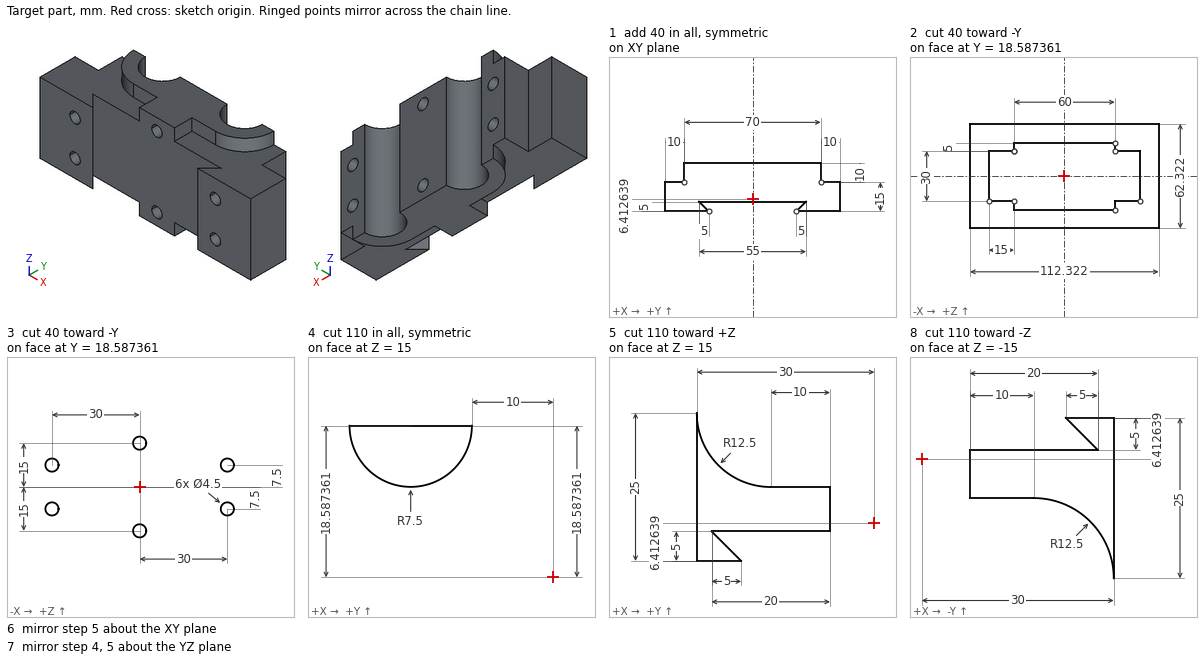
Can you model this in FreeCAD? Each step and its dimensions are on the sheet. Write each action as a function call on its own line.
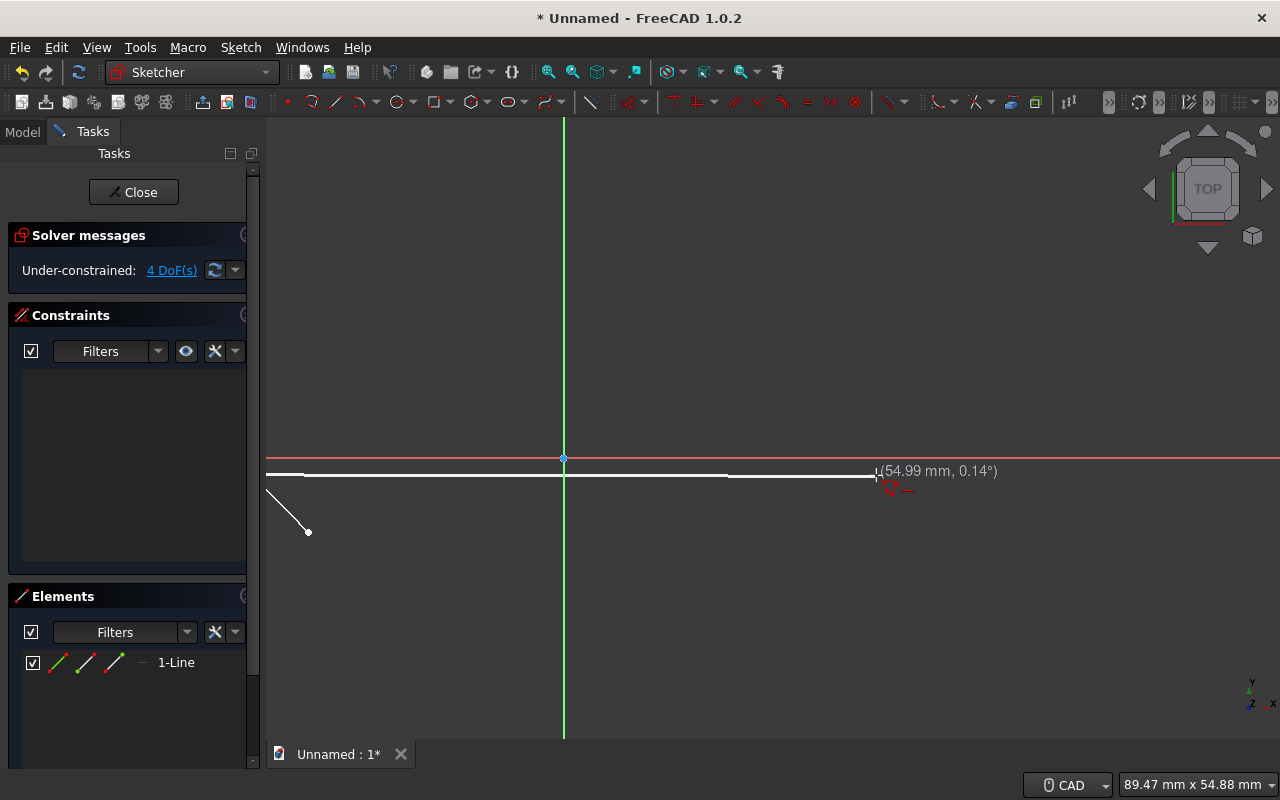
click(875, 474)
click(819, 531)
click(1074, 531)
click(1074, 361)
click(960, 361)
click(960, 247)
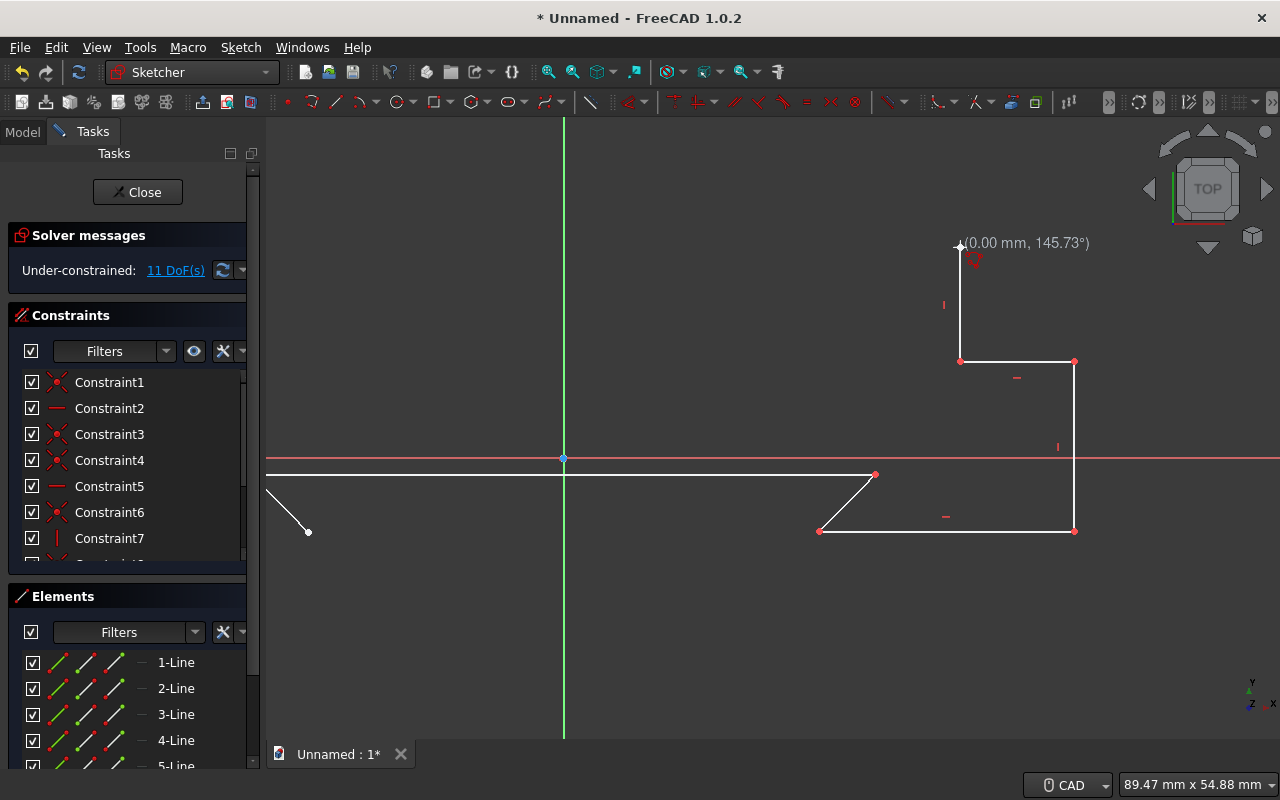
scroll(876, 475, down, 3)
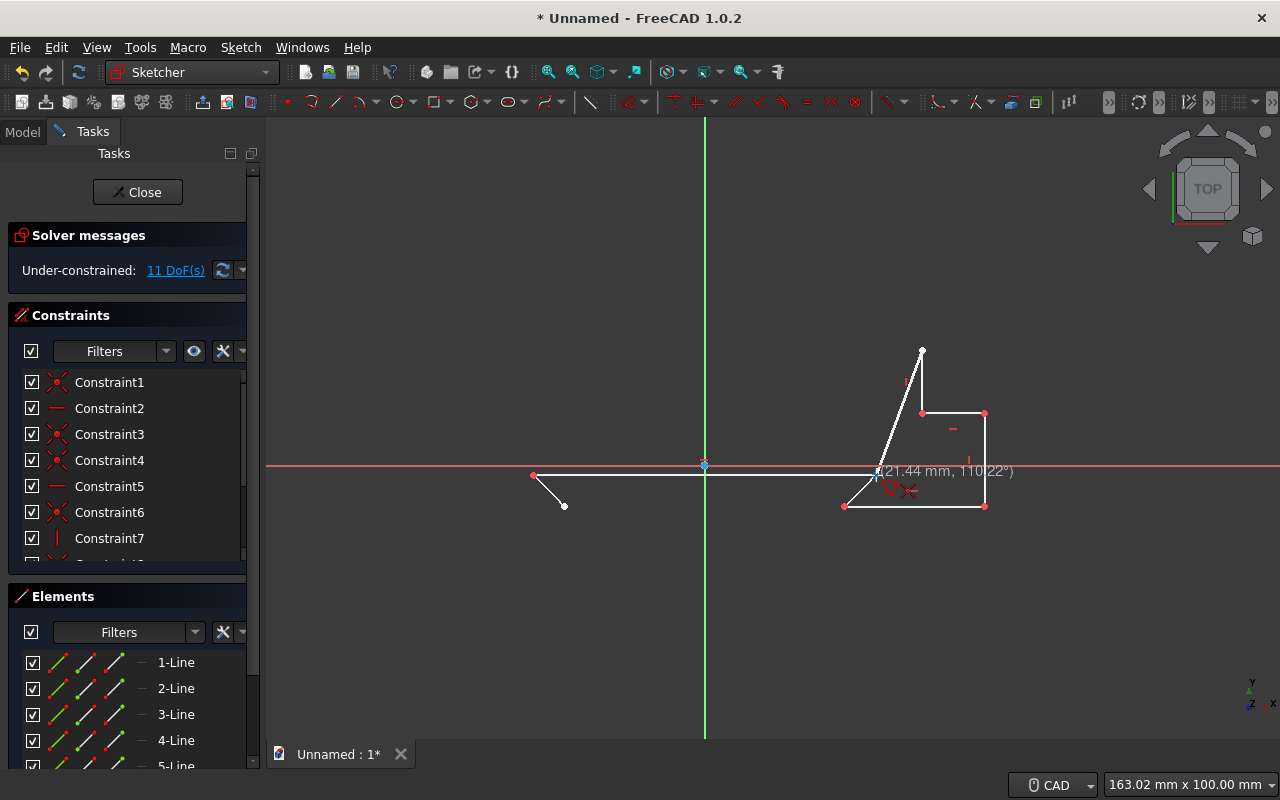
click(487, 350)
click(487, 413)
click(425, 413)
click(425, 506)
click(565, 507)
key(Escape)
key(Escape)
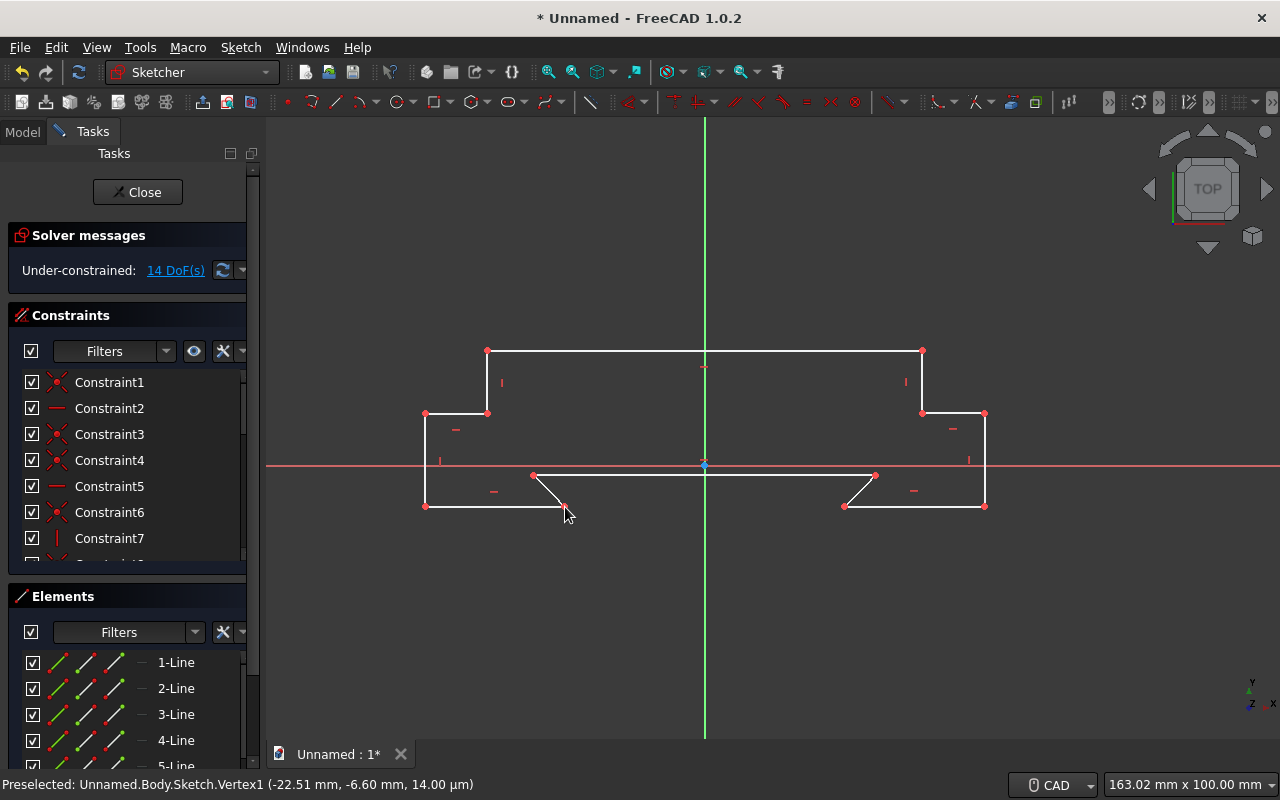
click(565, 507)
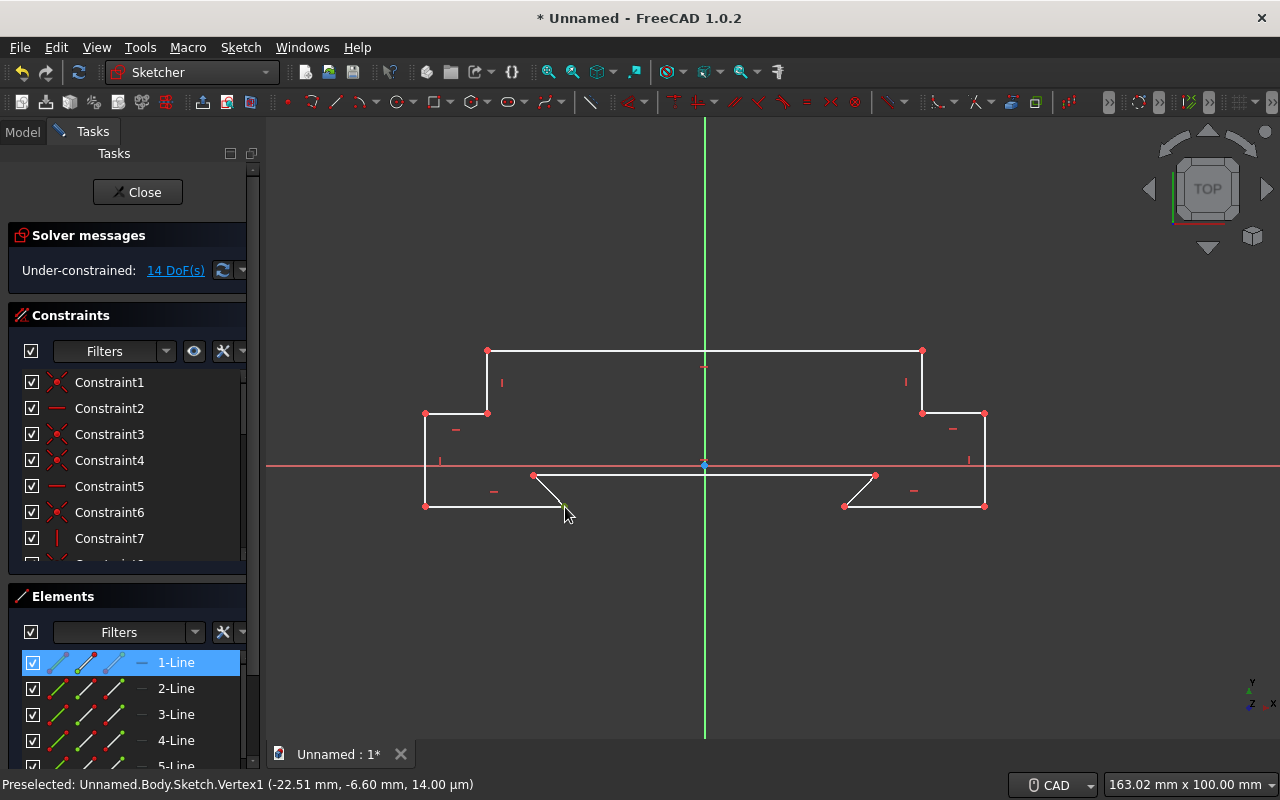
click(845, 507)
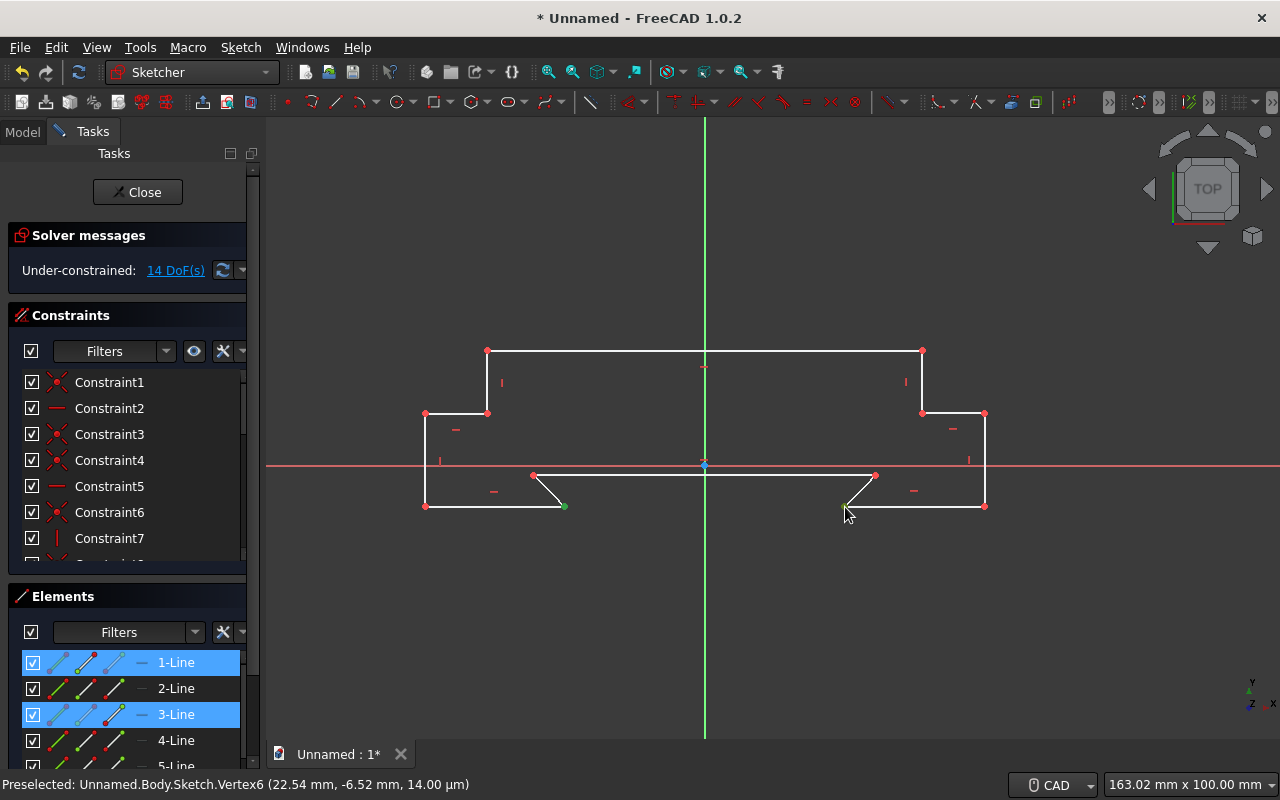
click(705, 671)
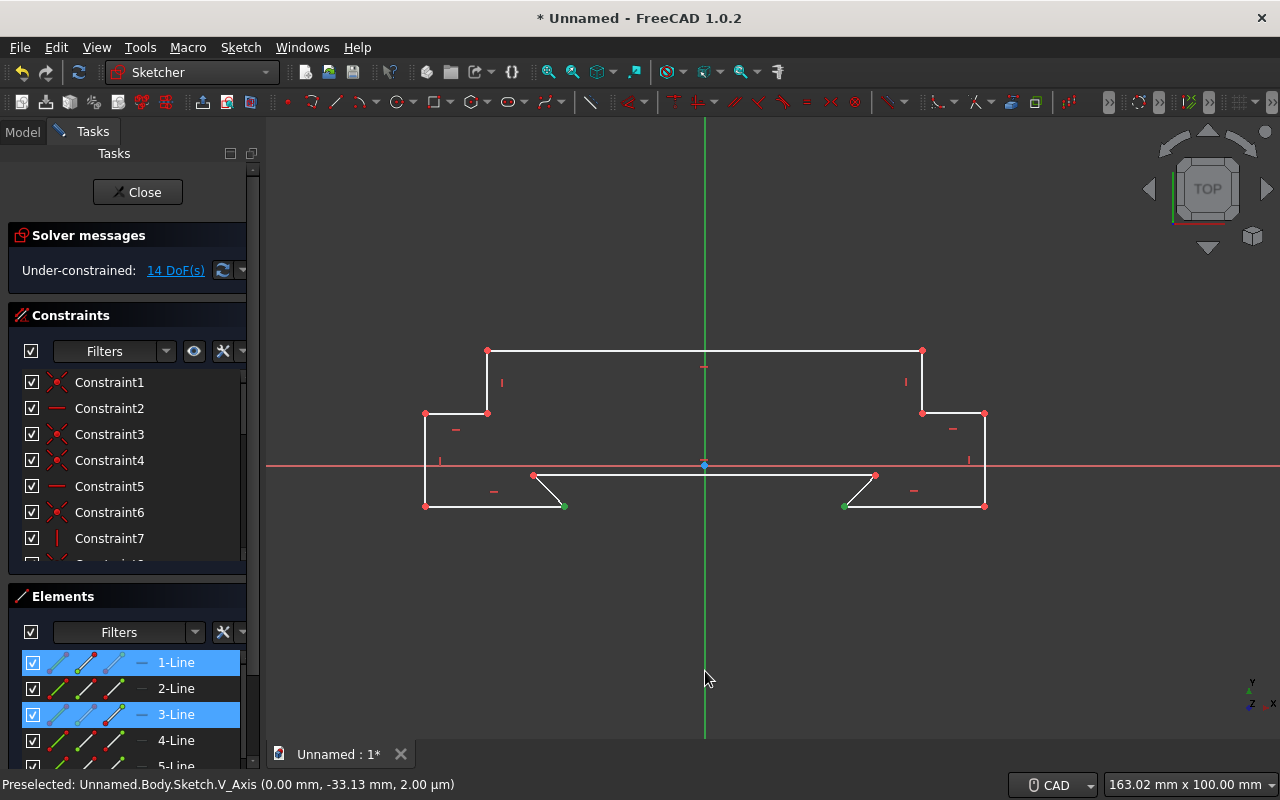
key(s)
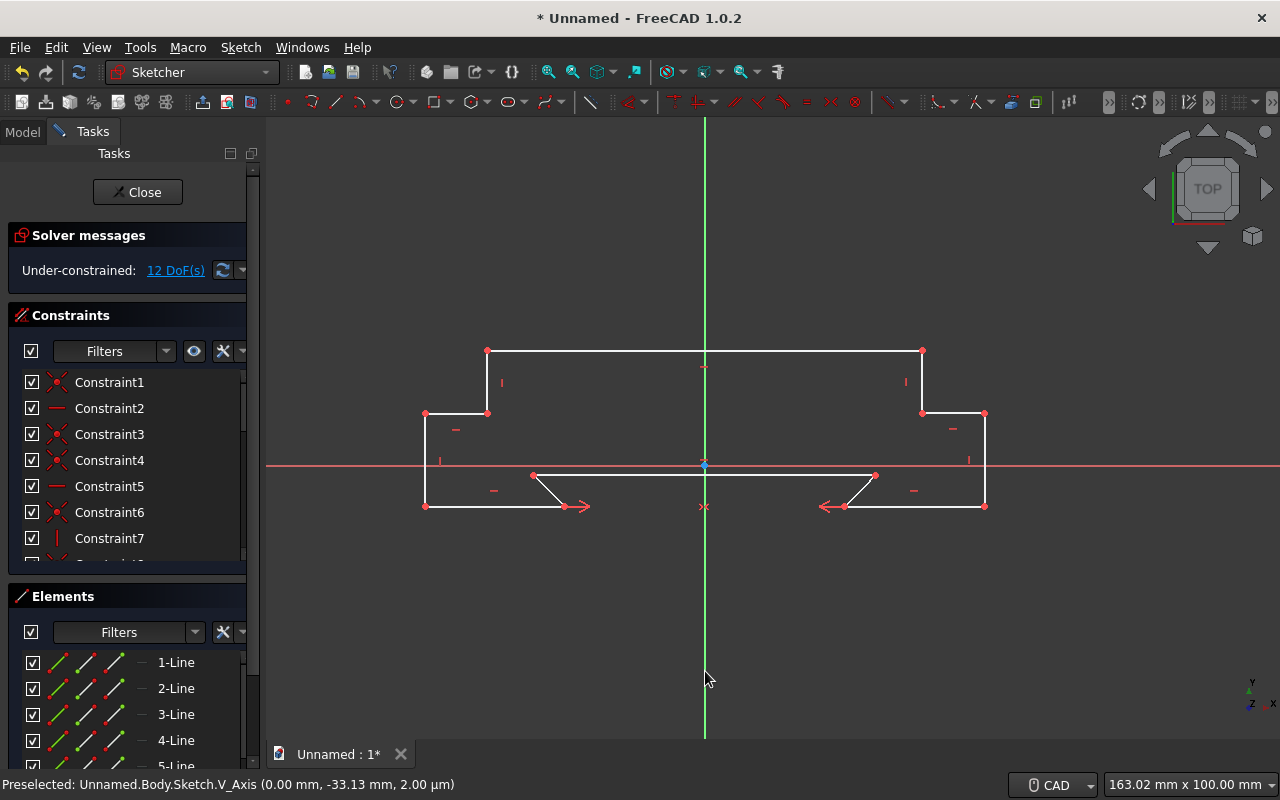
click(922, 413)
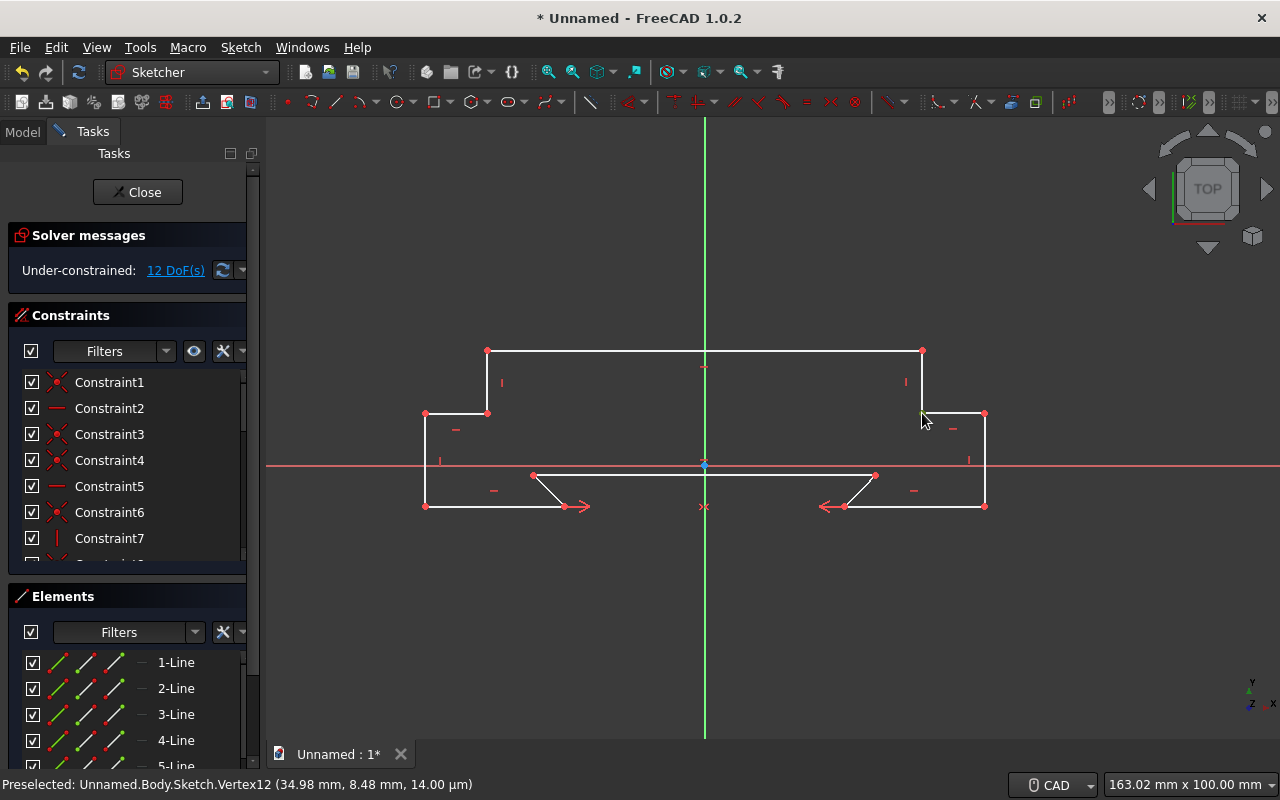
click(487, 414)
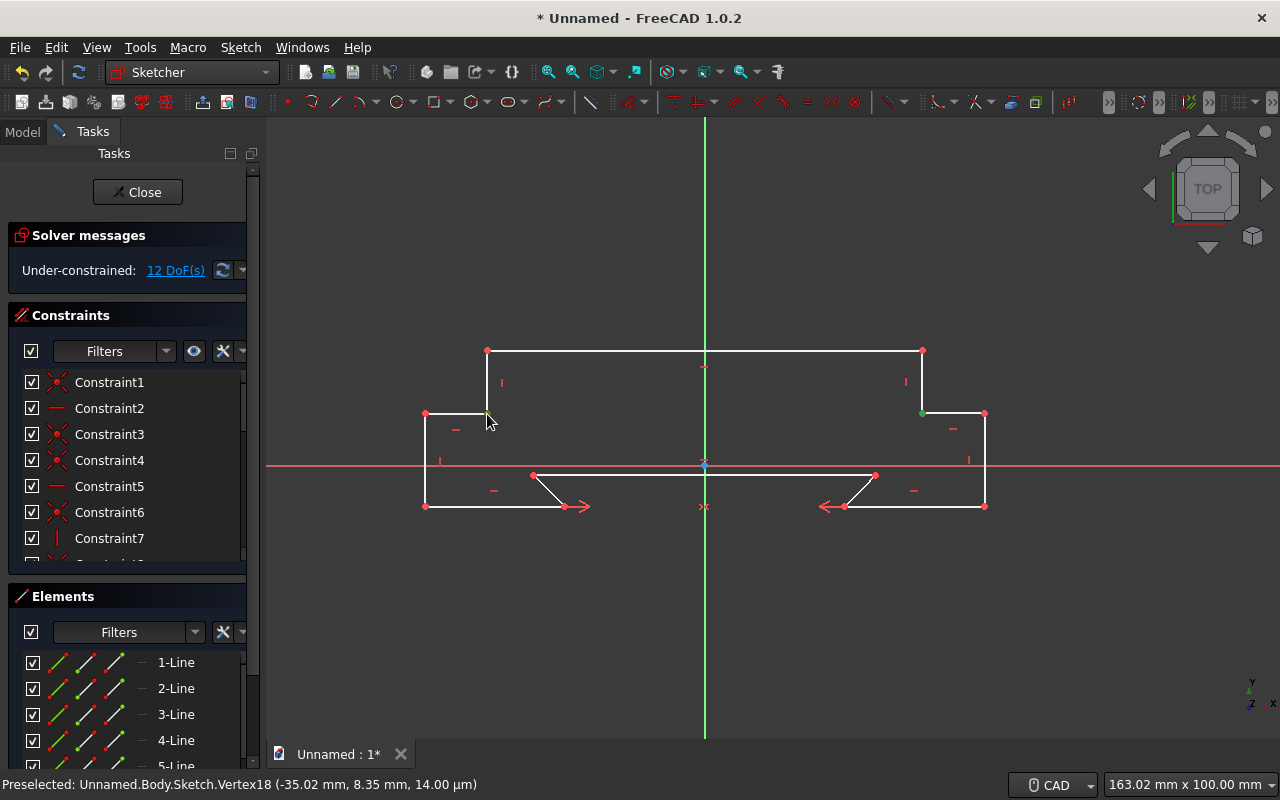
click(705, 671)